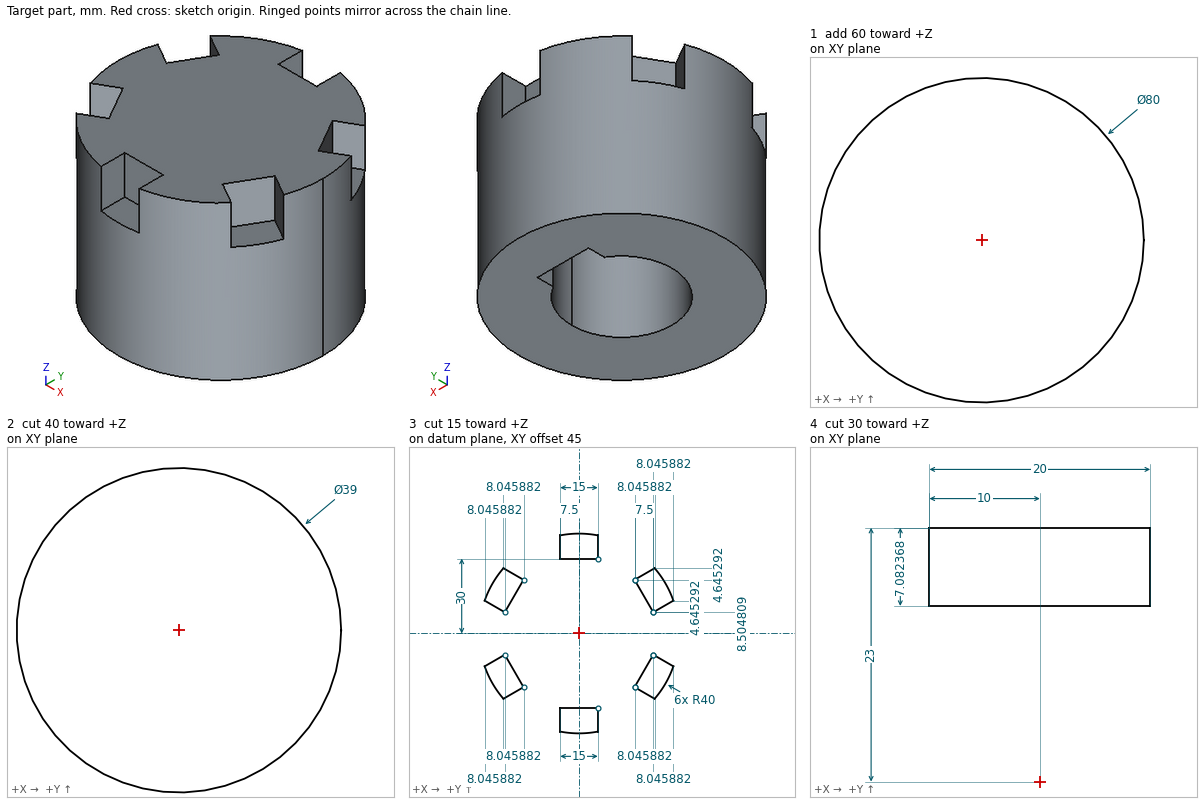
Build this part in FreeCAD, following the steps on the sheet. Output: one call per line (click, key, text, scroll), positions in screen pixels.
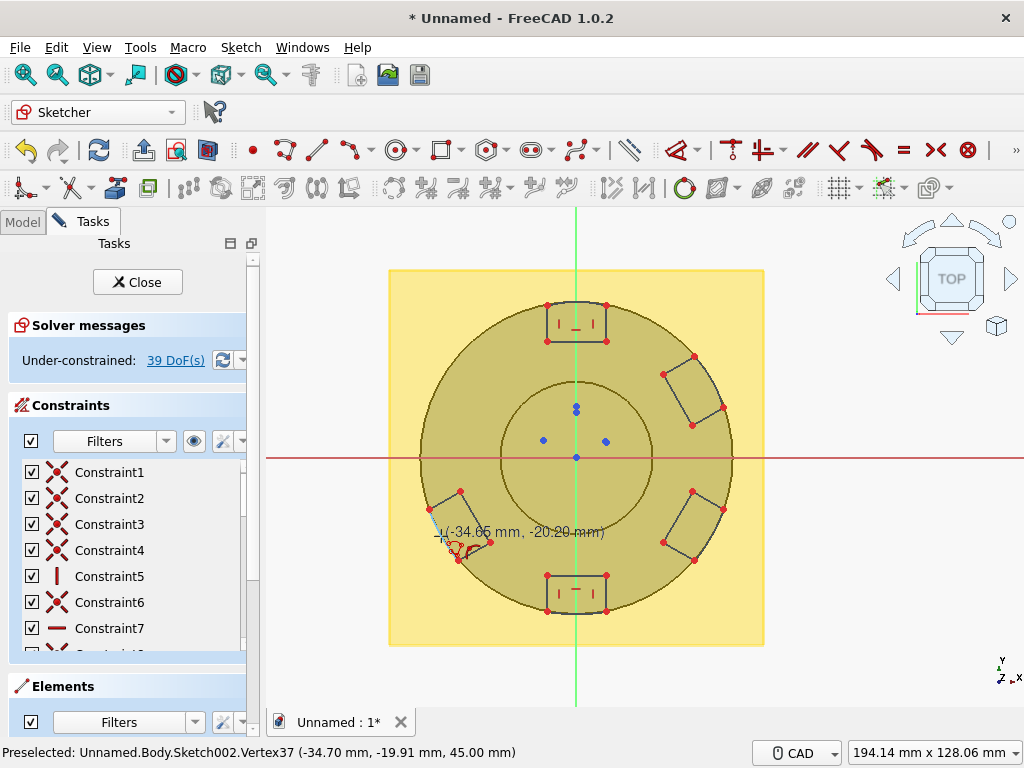
click(429, 406)
click(460, 425)
click(490, 374)
click(458, 356)
right_click(458, 356)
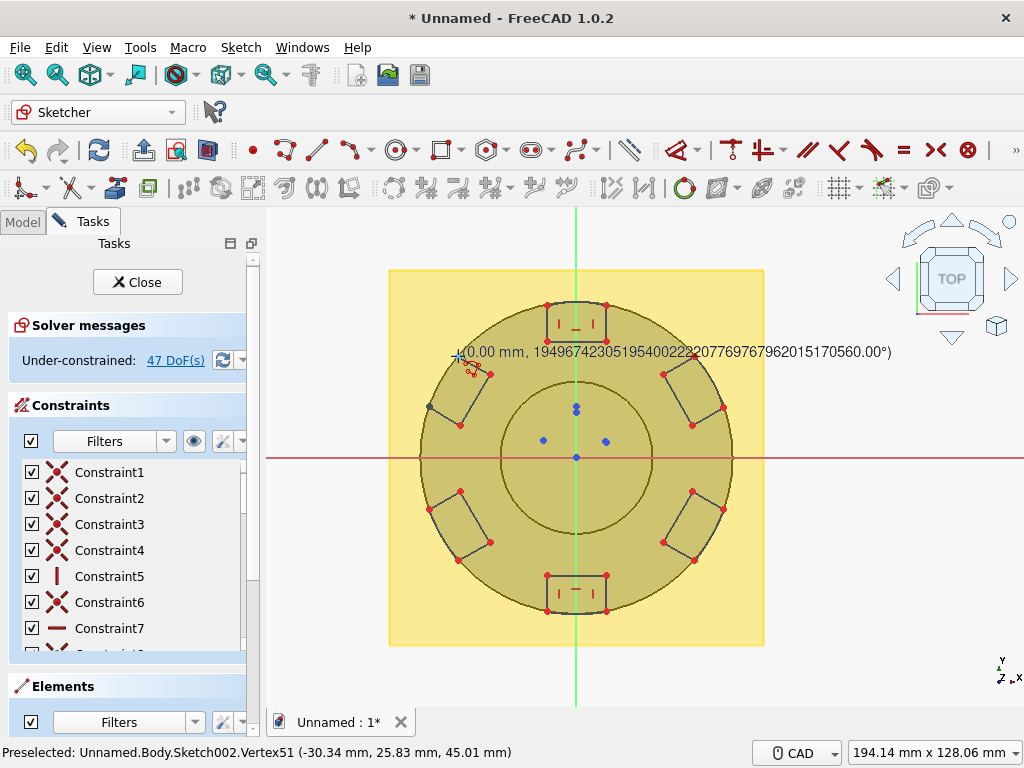
click(350, 150)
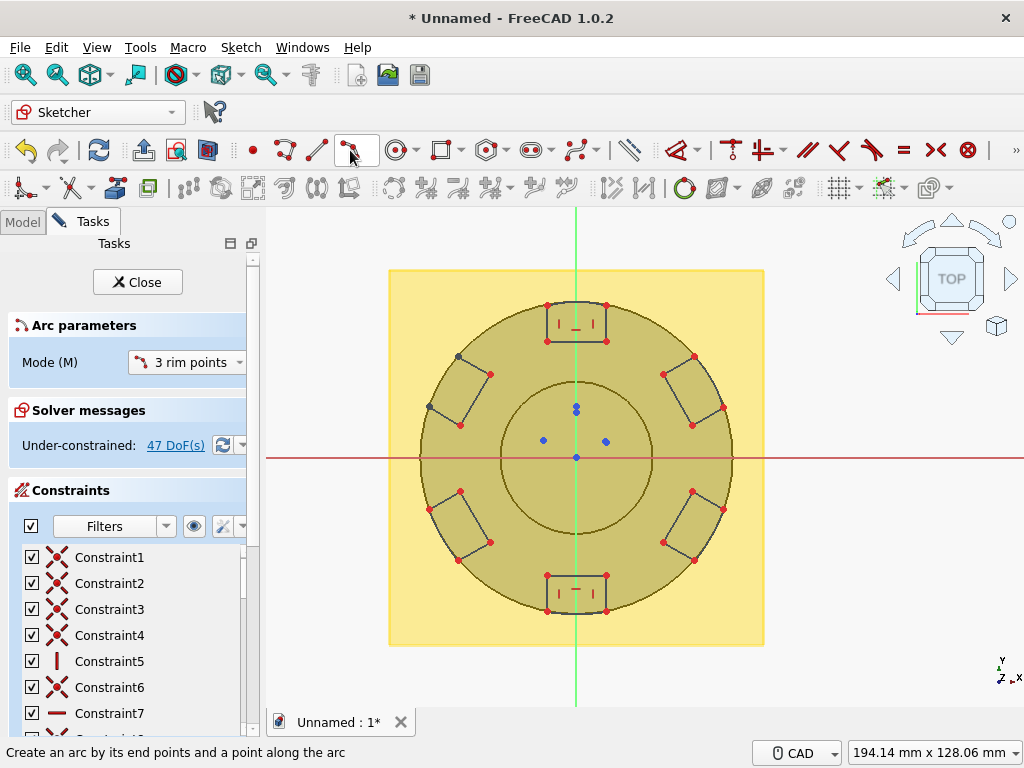
click(458, 357)
click(429, 407)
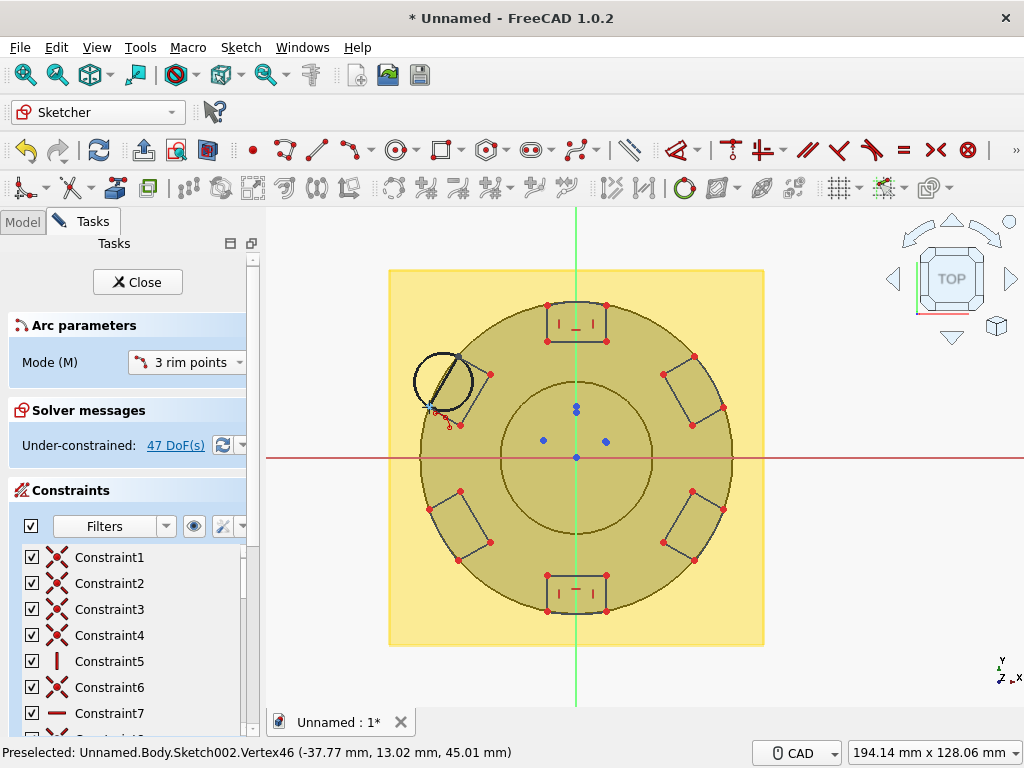
scroll(441, 380, up, 9)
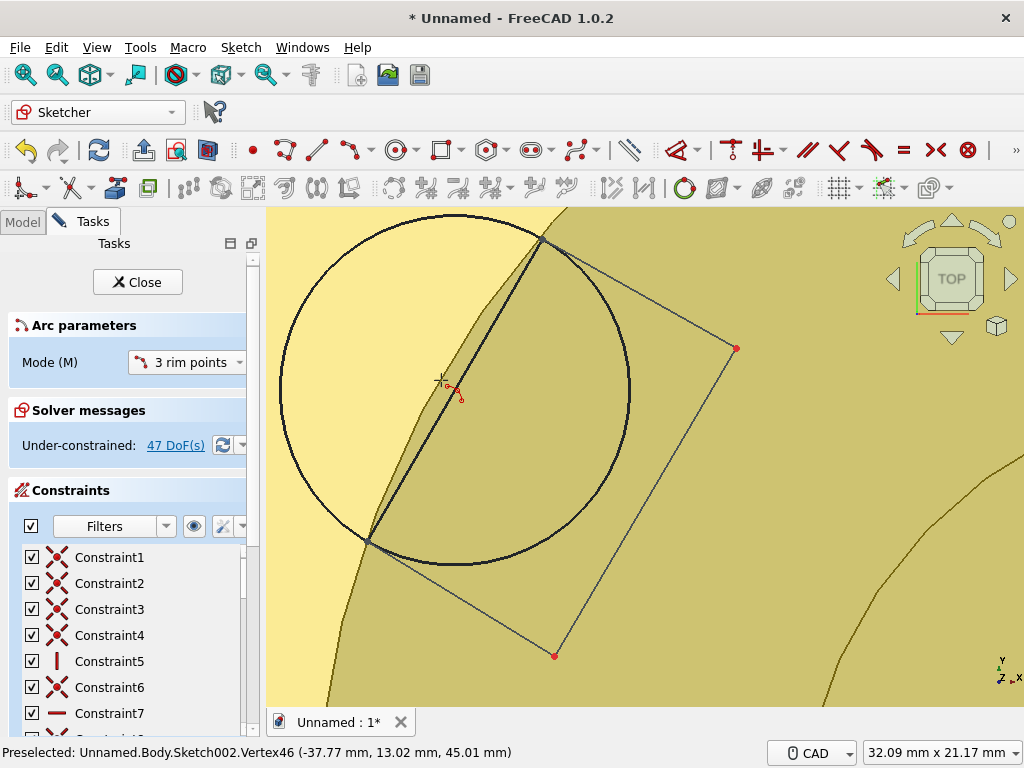
click(441, 377)
key(Escape)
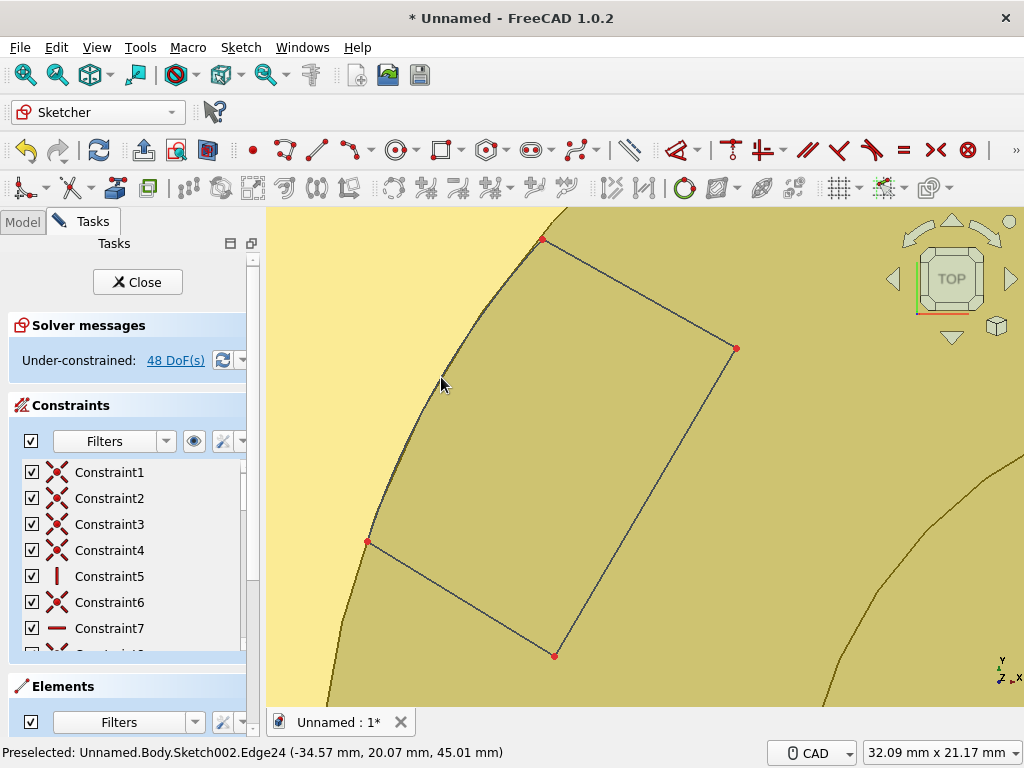
scroll(441, 379, down, 9)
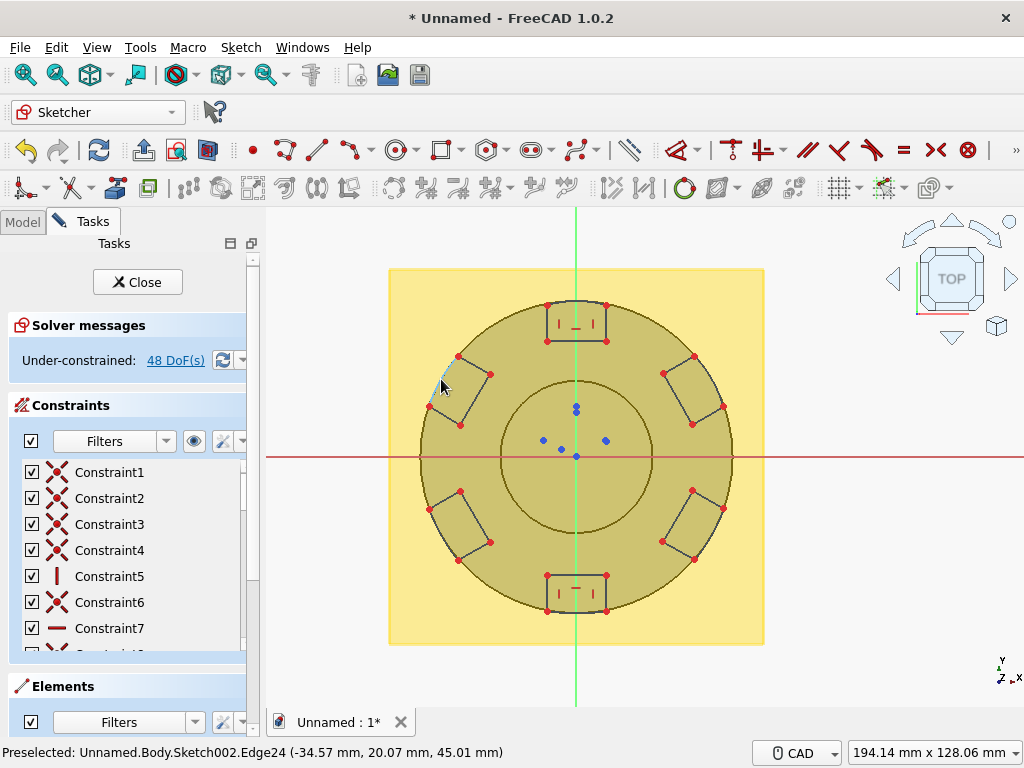
click(717, 390)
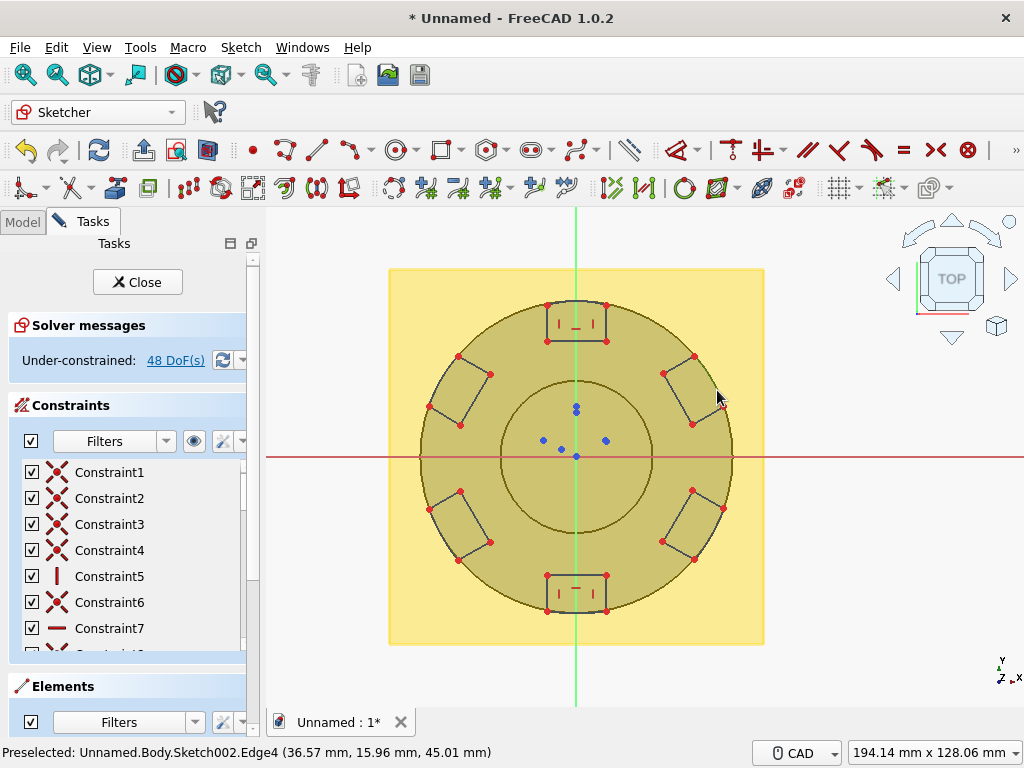
click(589, 302)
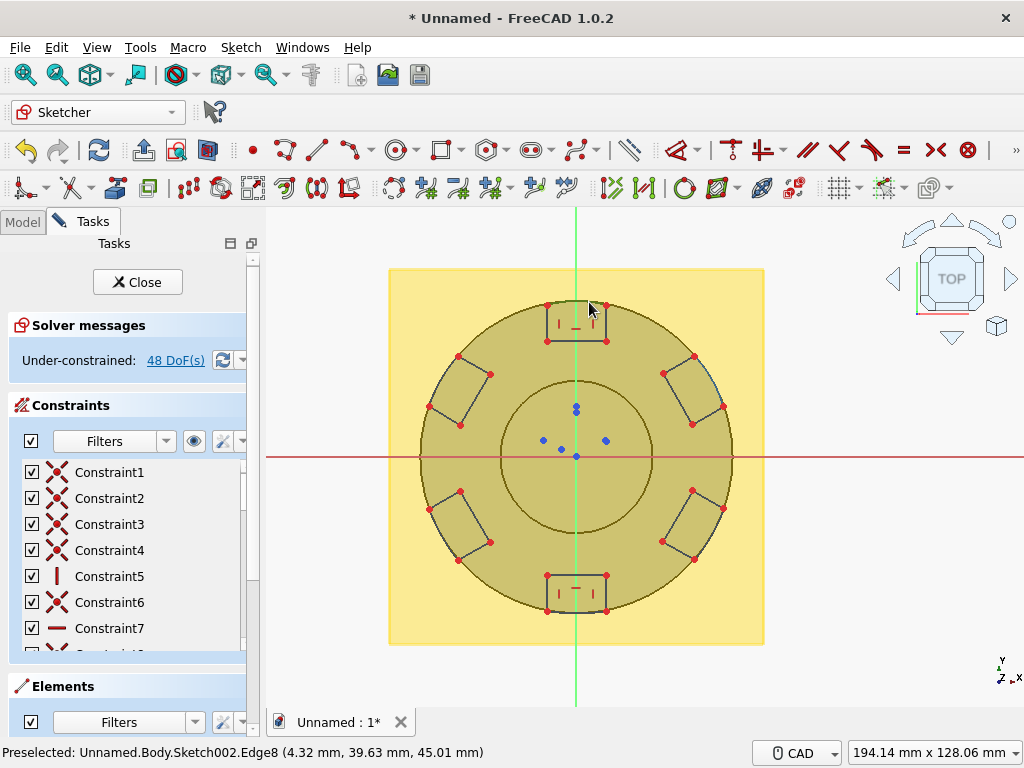
click(732, 150)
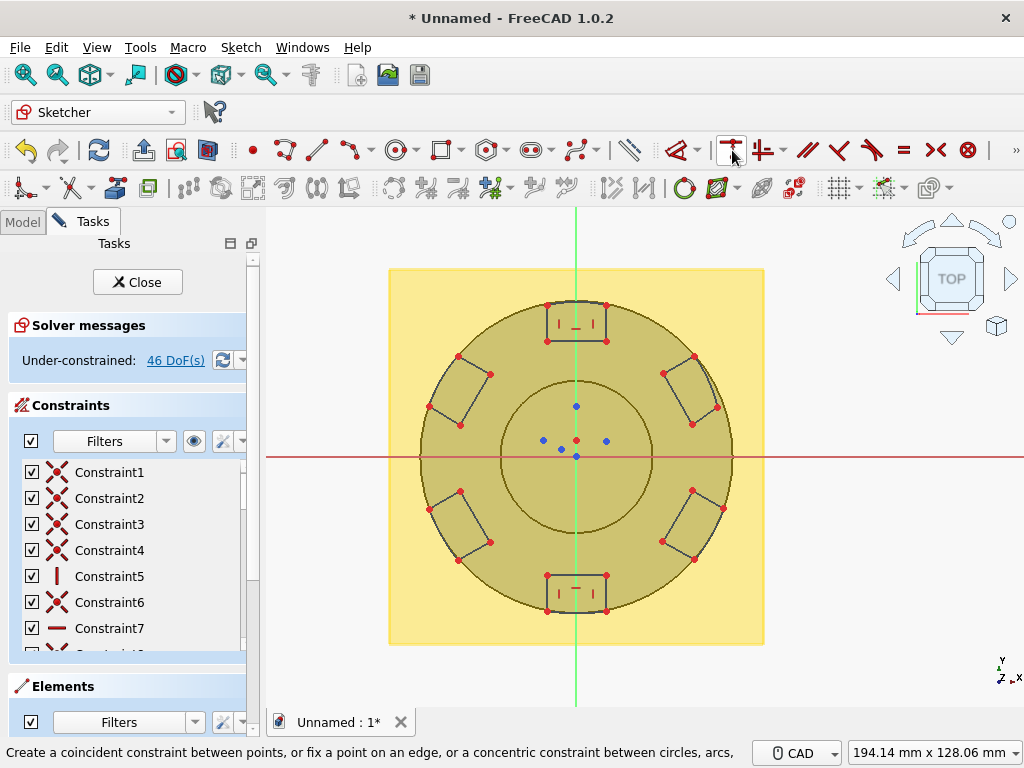
click(713, 391)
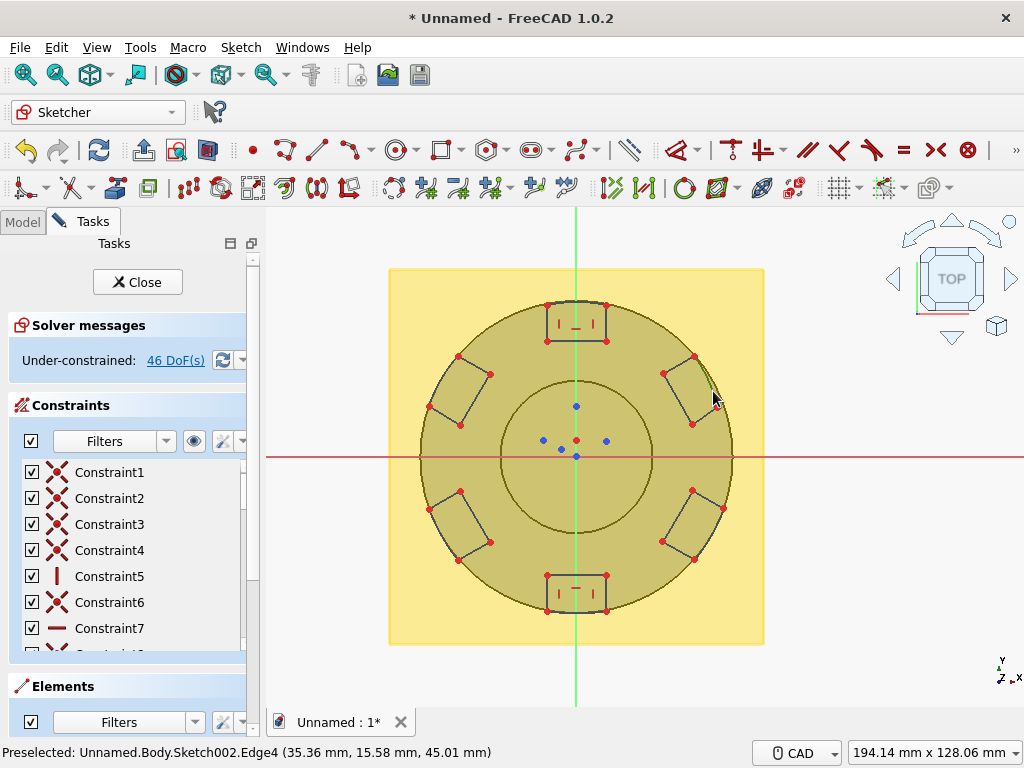
click(705, 546)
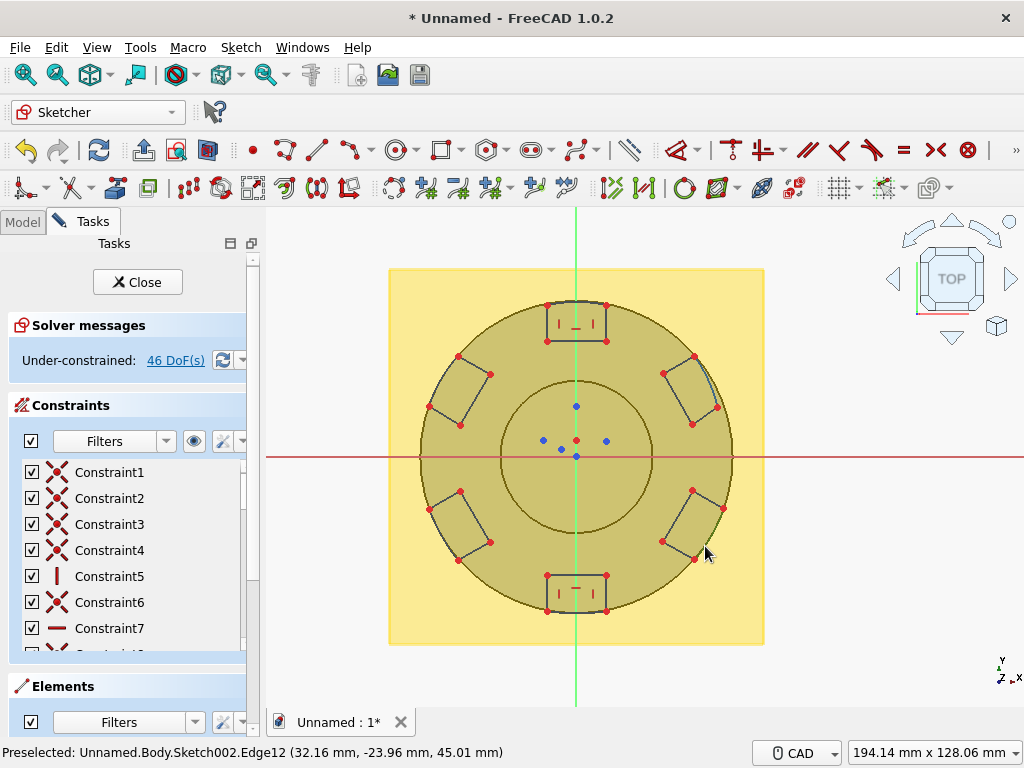
click(732, 150)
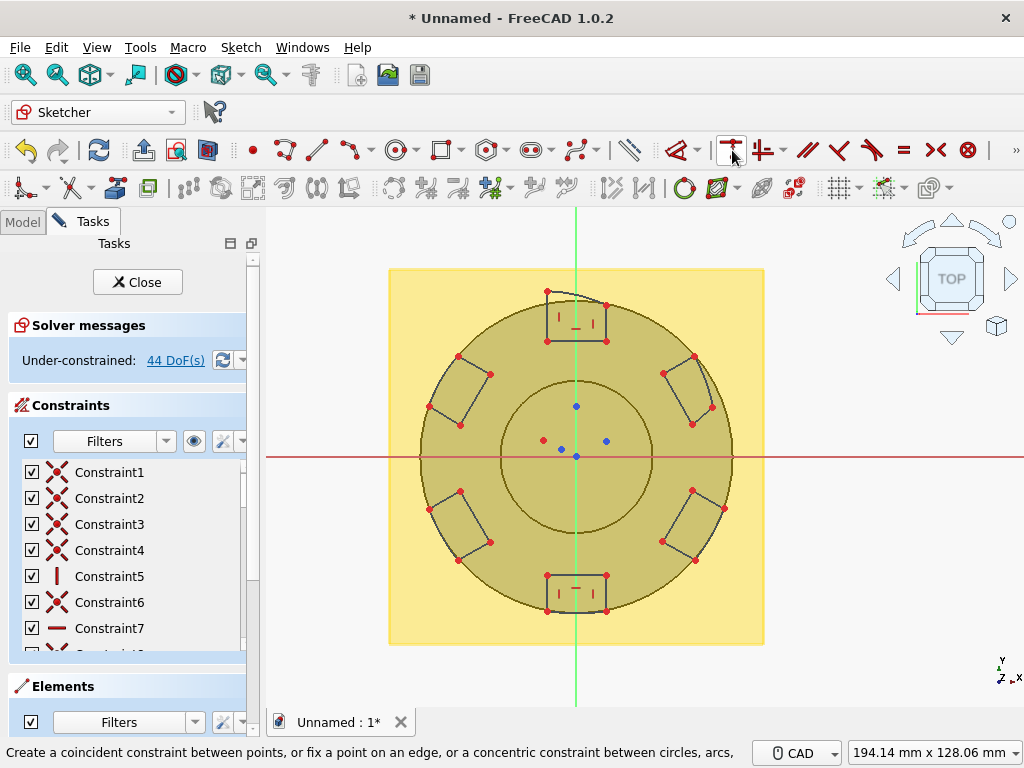
click(709, 391)